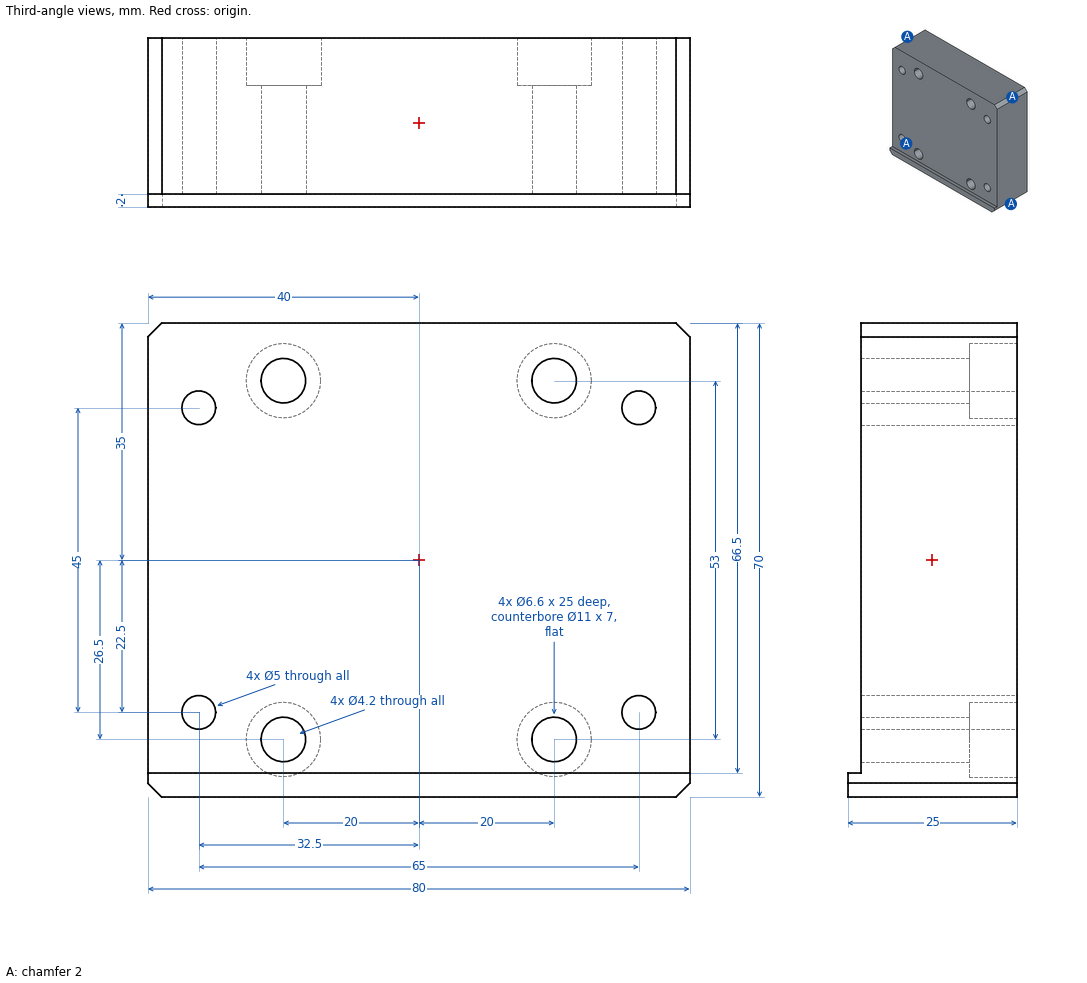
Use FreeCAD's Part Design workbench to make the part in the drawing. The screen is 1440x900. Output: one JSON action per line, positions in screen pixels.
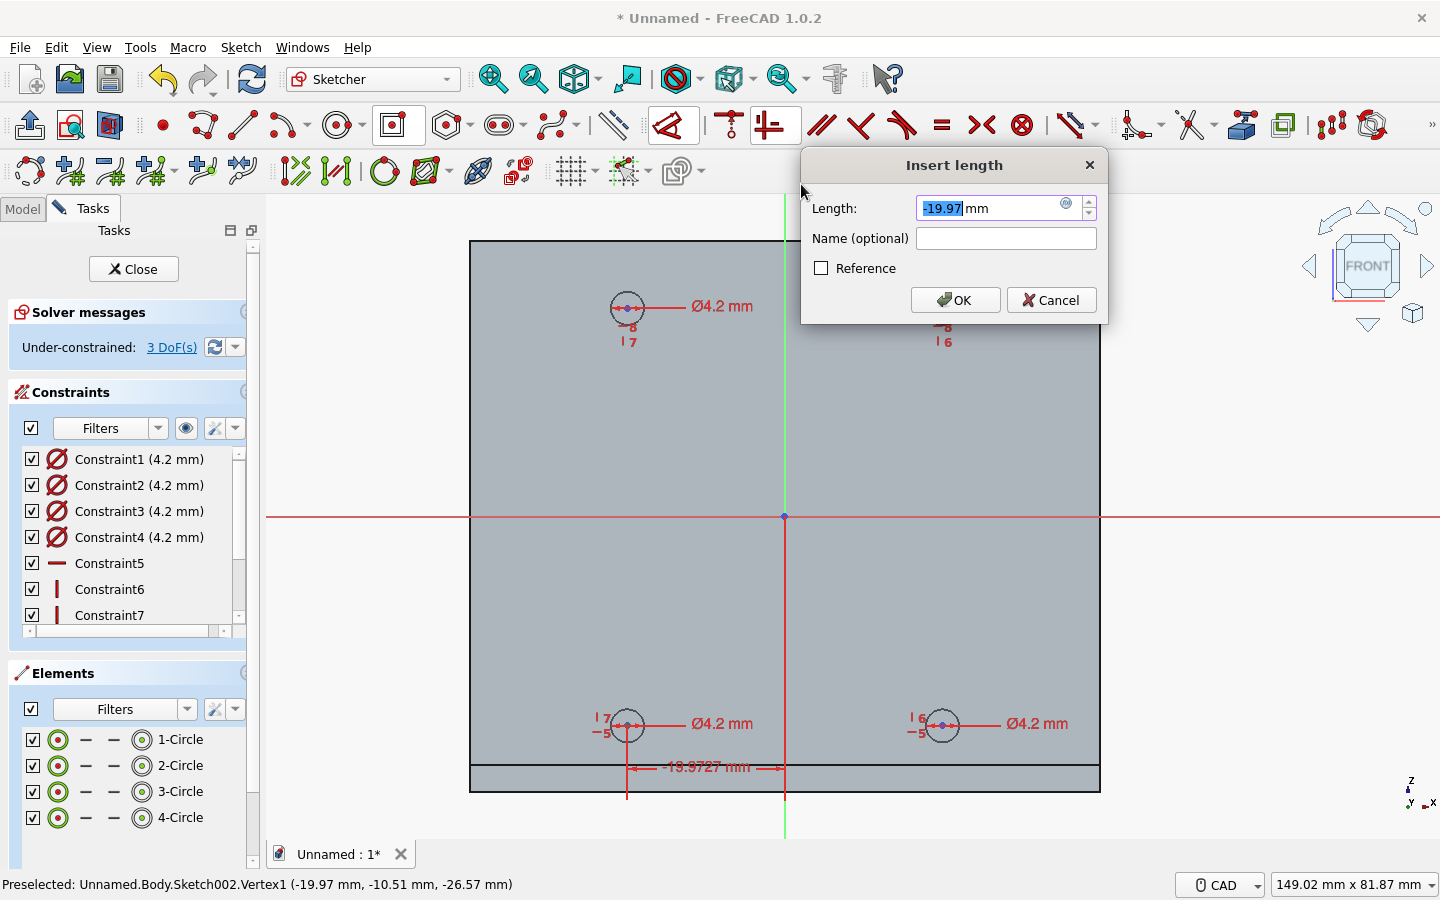
{"action": "type", "text": "-20"}
{"action": "key", "text": "Return"}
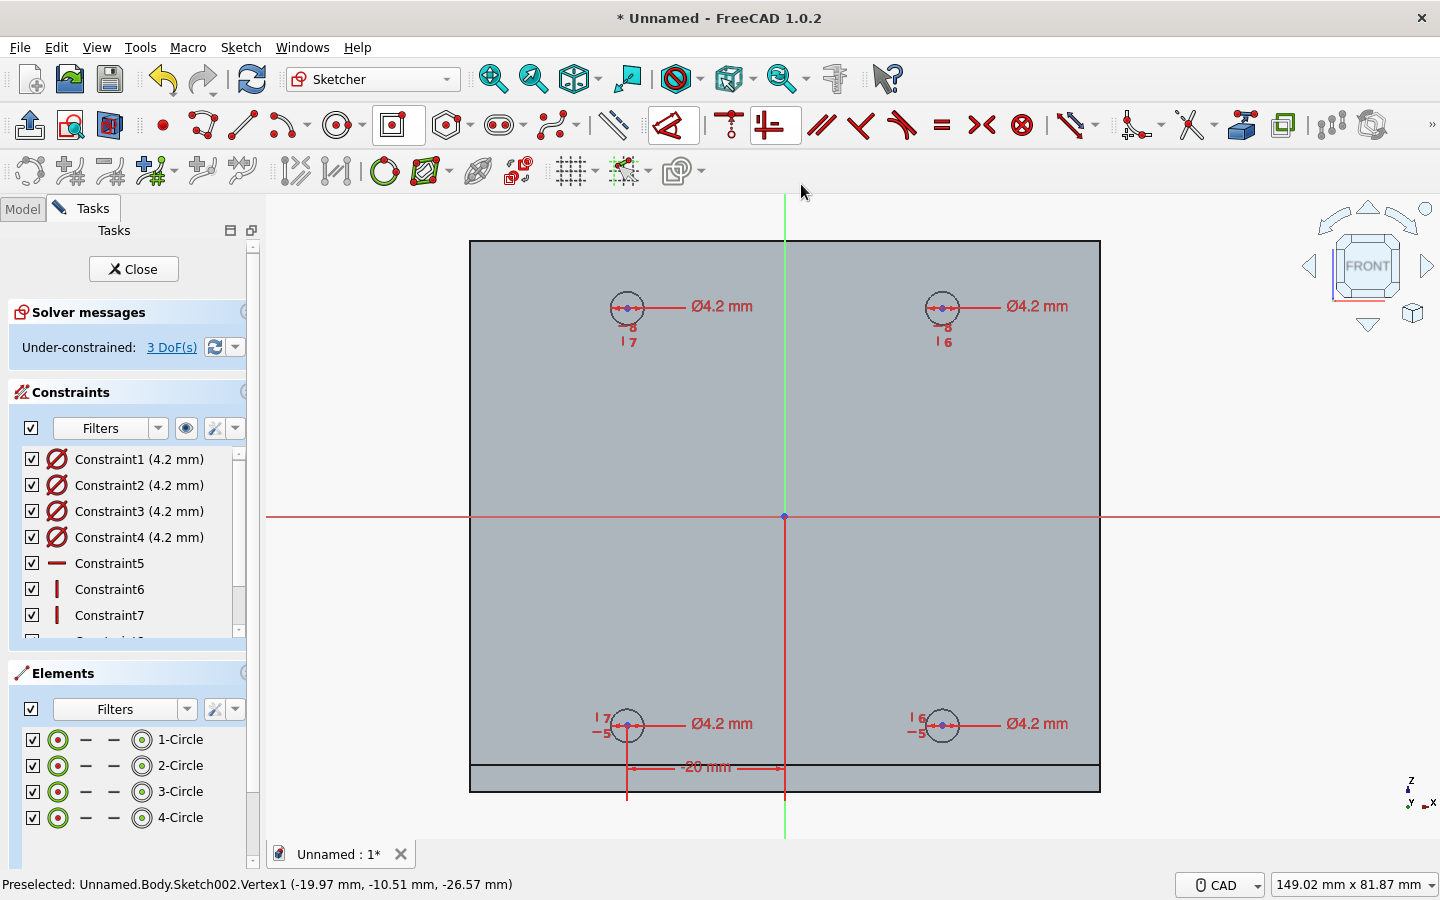
{"action": "left_click", "coordinate": [943, 726]}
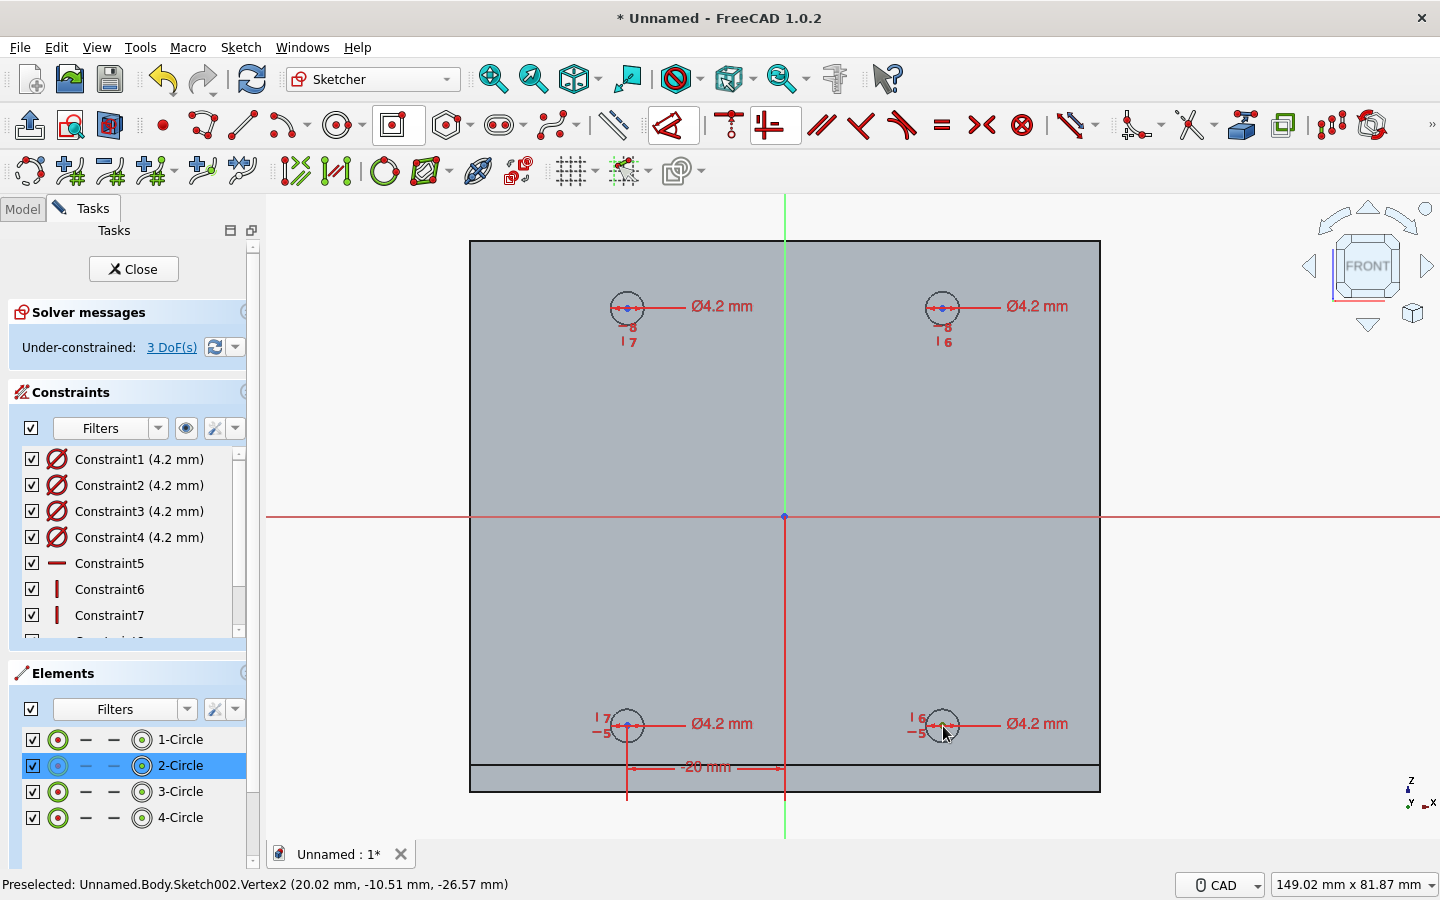
{"action": "key", "text": "l"}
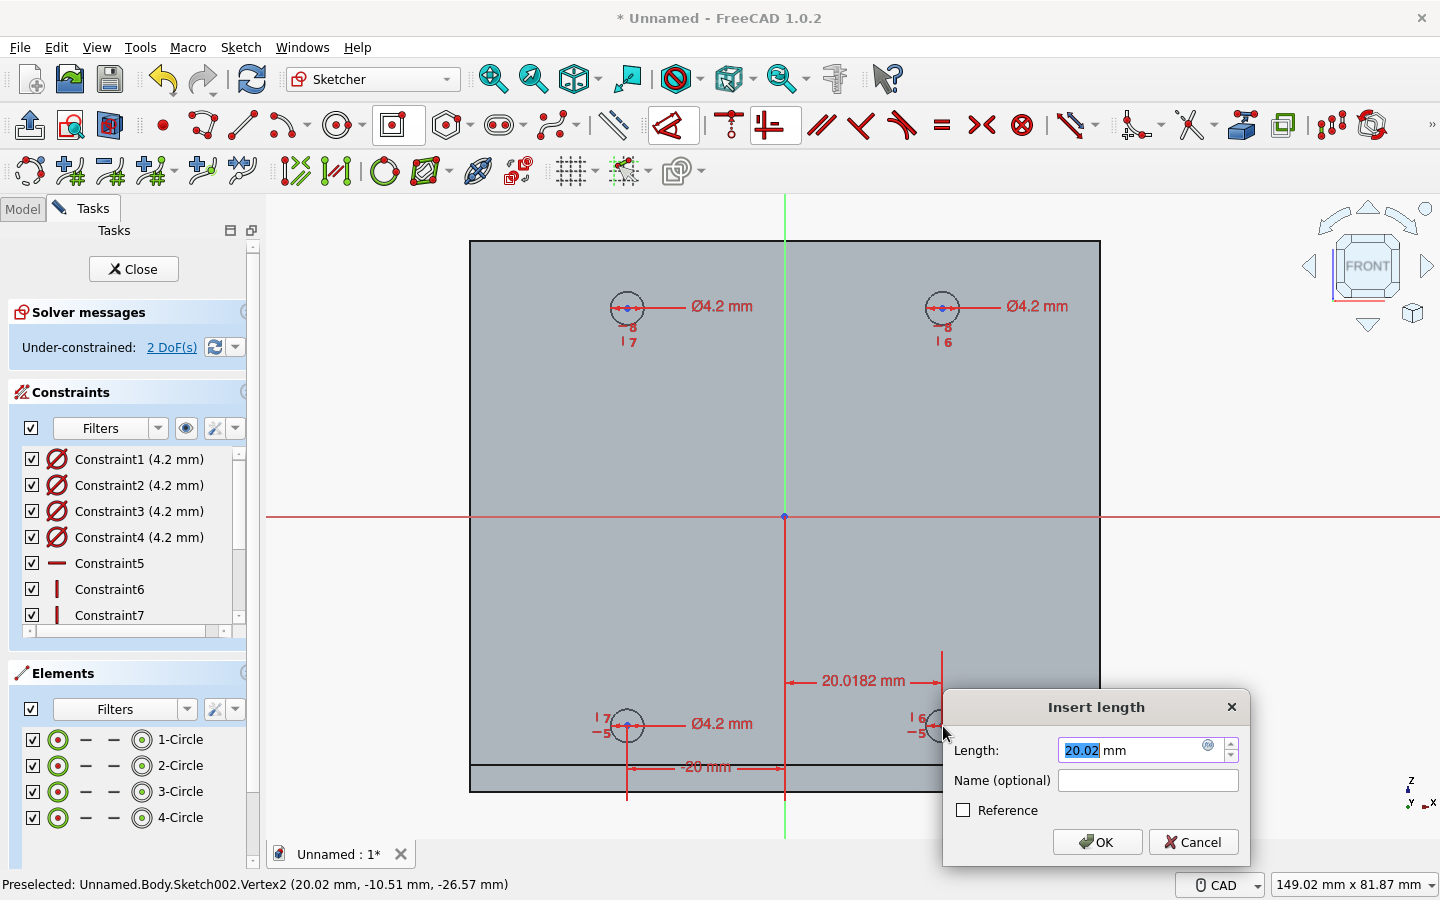
{"action": "type", "text": "20"}
{"action": "key", "text": "Return"}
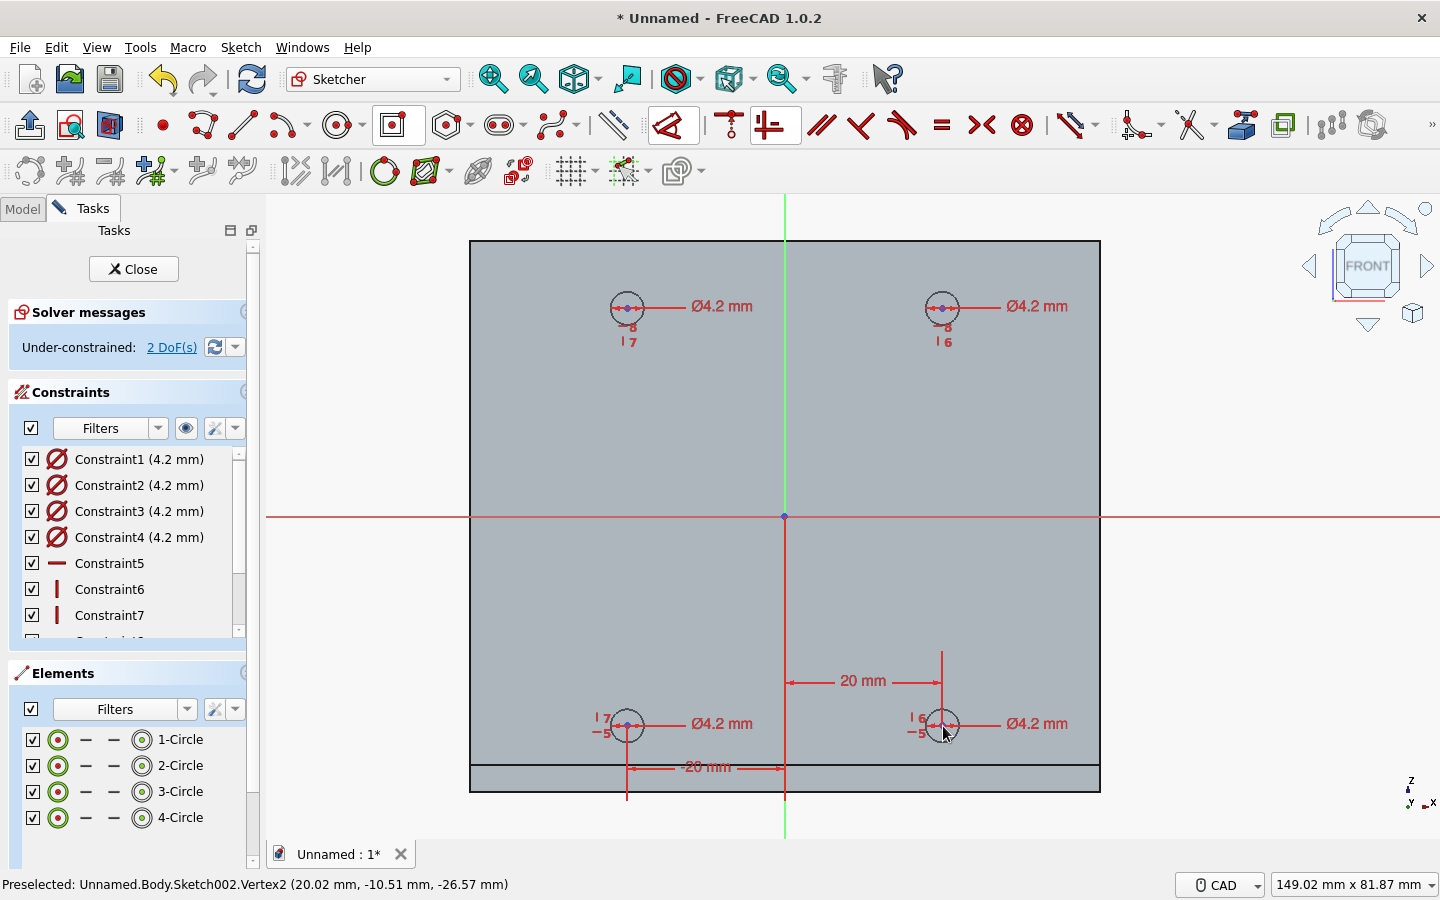
{"action": "left_click", "coordinate": [942, 726]}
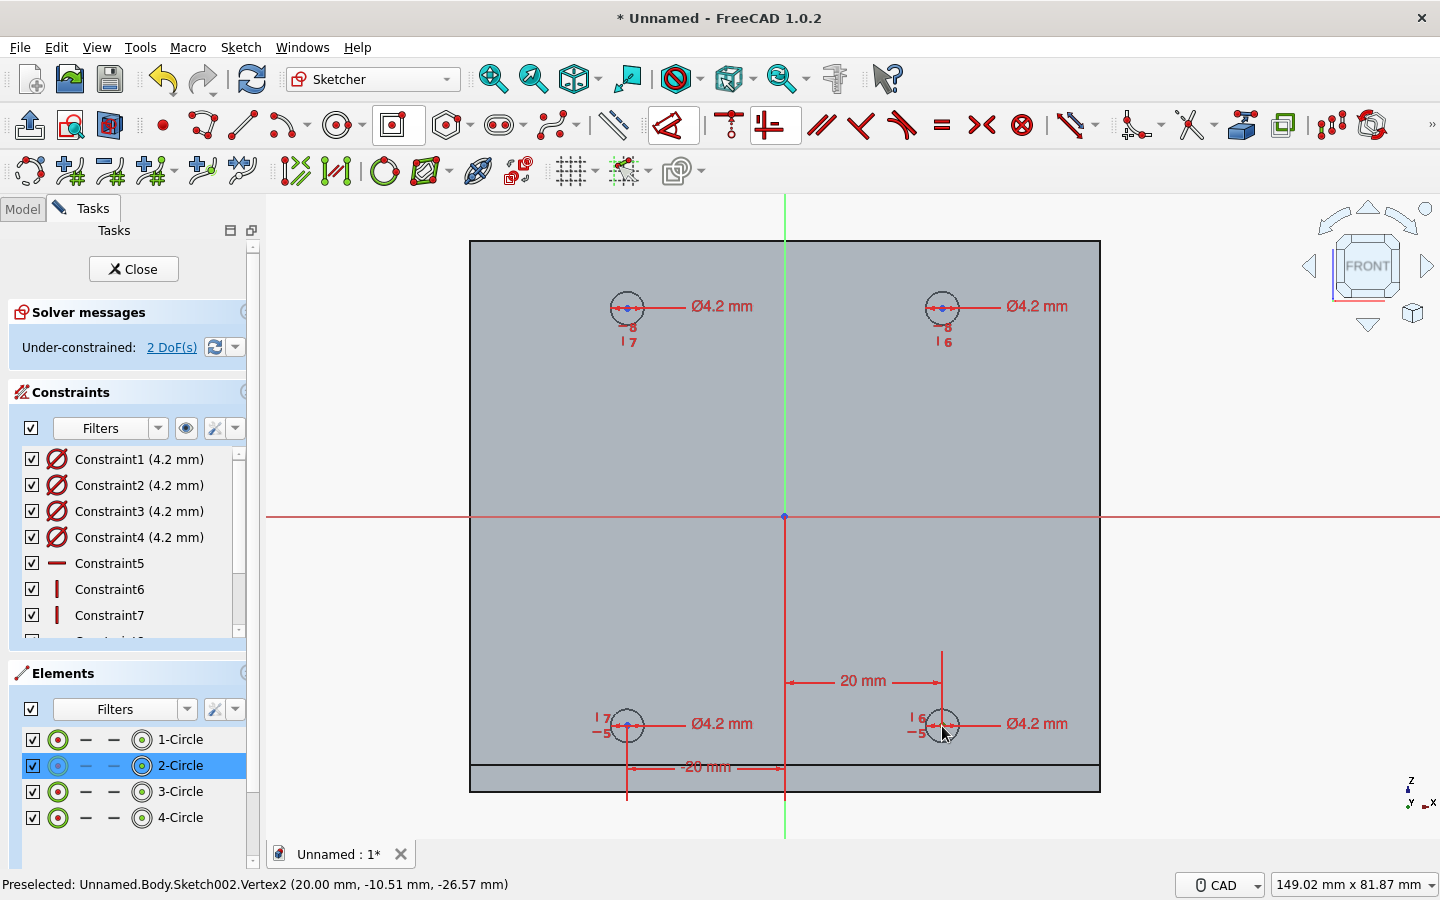
{"action": "left_click", "coordinate": [942, 308]}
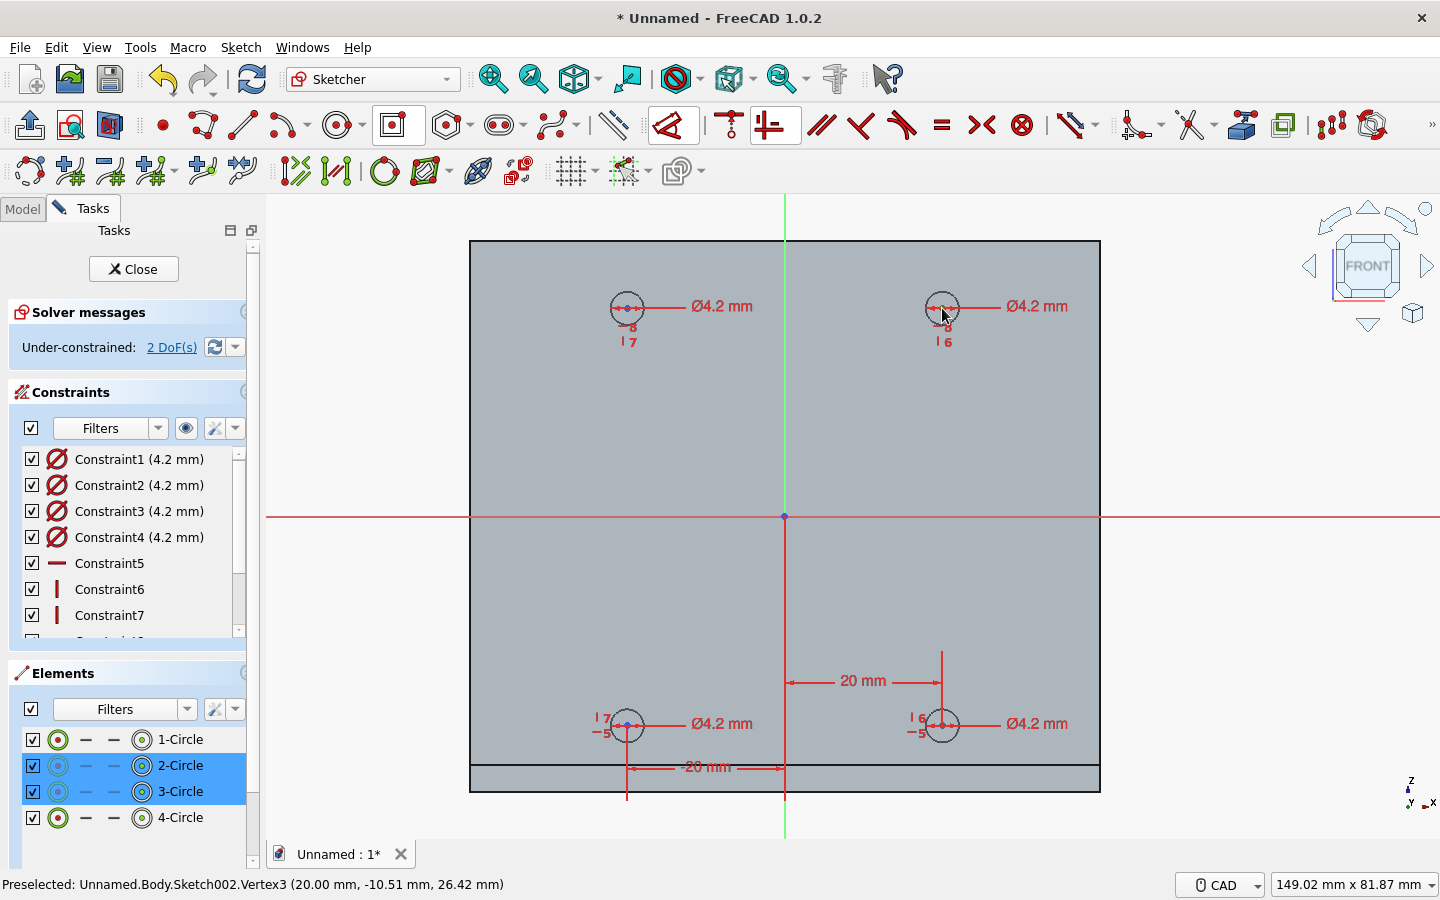
{"action": "key", "text": "i"}